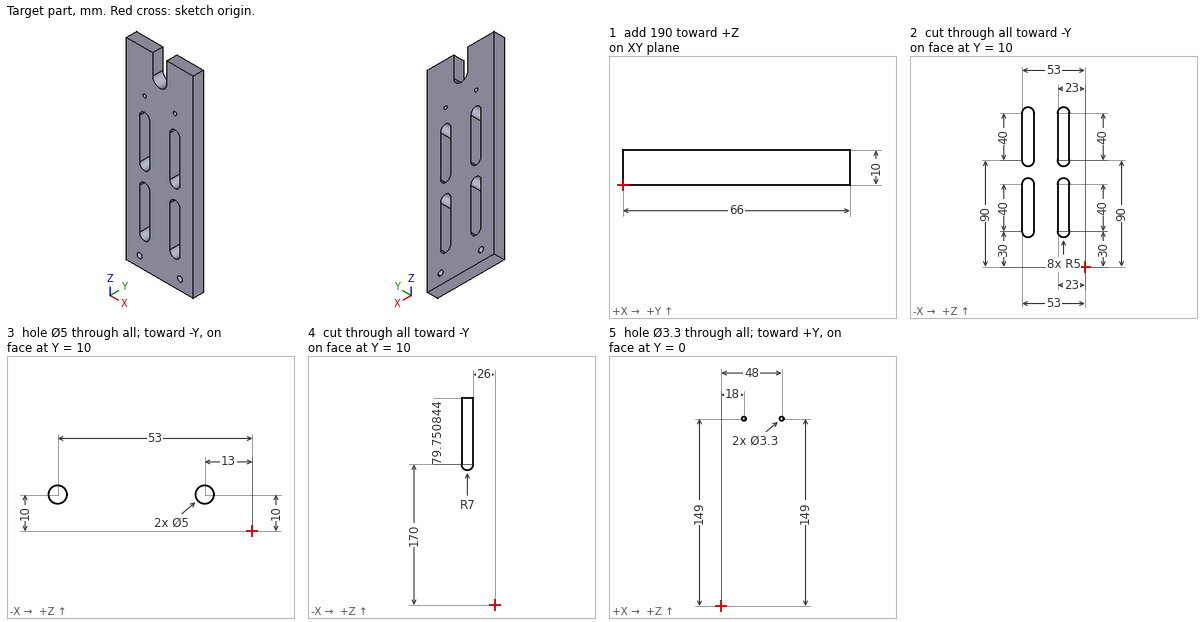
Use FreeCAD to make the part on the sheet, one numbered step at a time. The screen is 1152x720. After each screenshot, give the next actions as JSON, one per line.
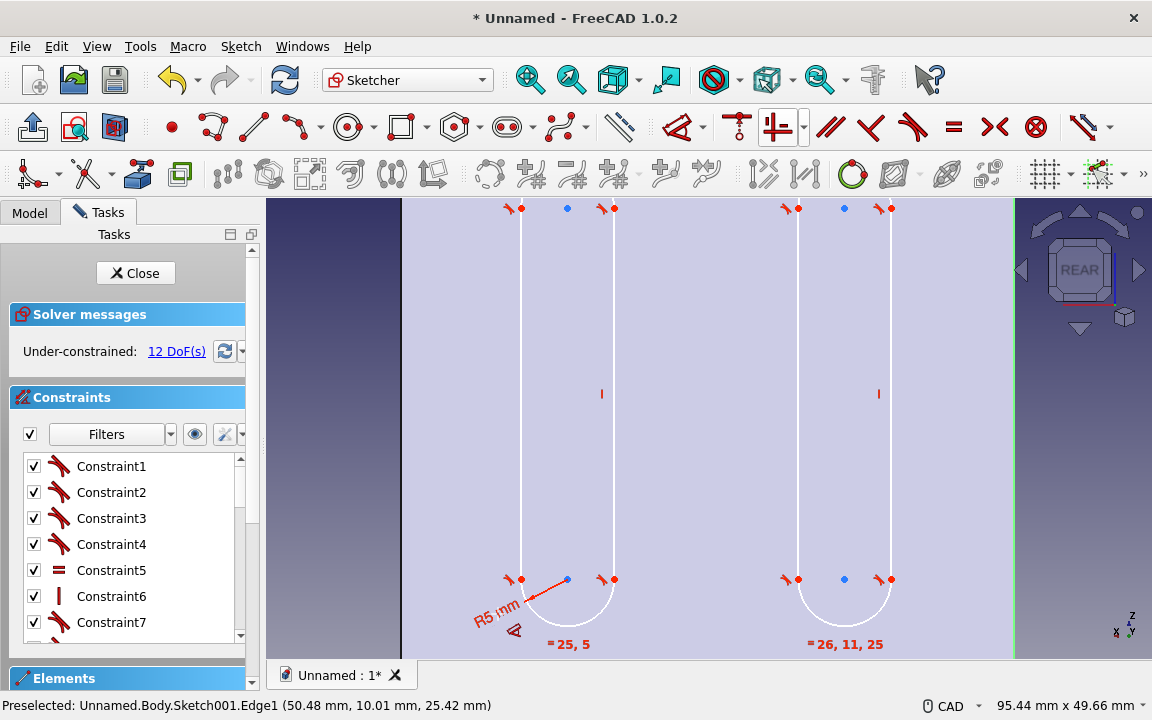
{"action": "scroll", "coordinate": [599, 494], "scroll_direction": "down", "scroll_amount": 7}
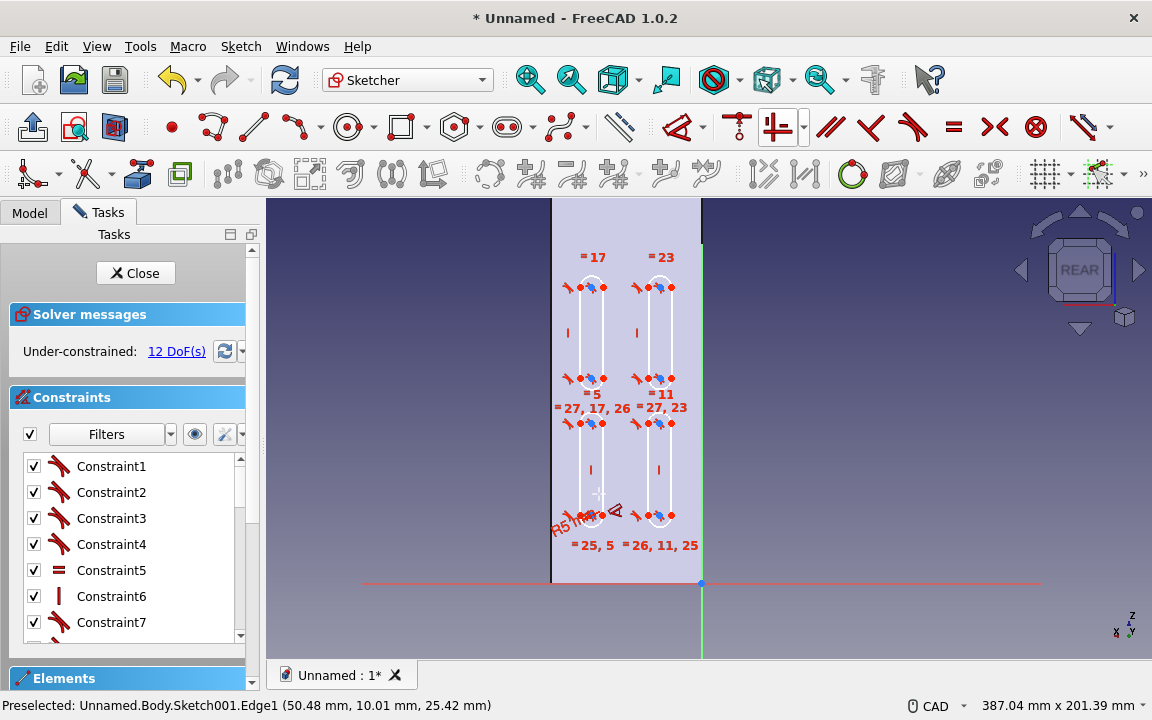
{"action": "left_click", "coordinate": [580, 488]}
{"action": "left_click", "coordinate": [546, 470]}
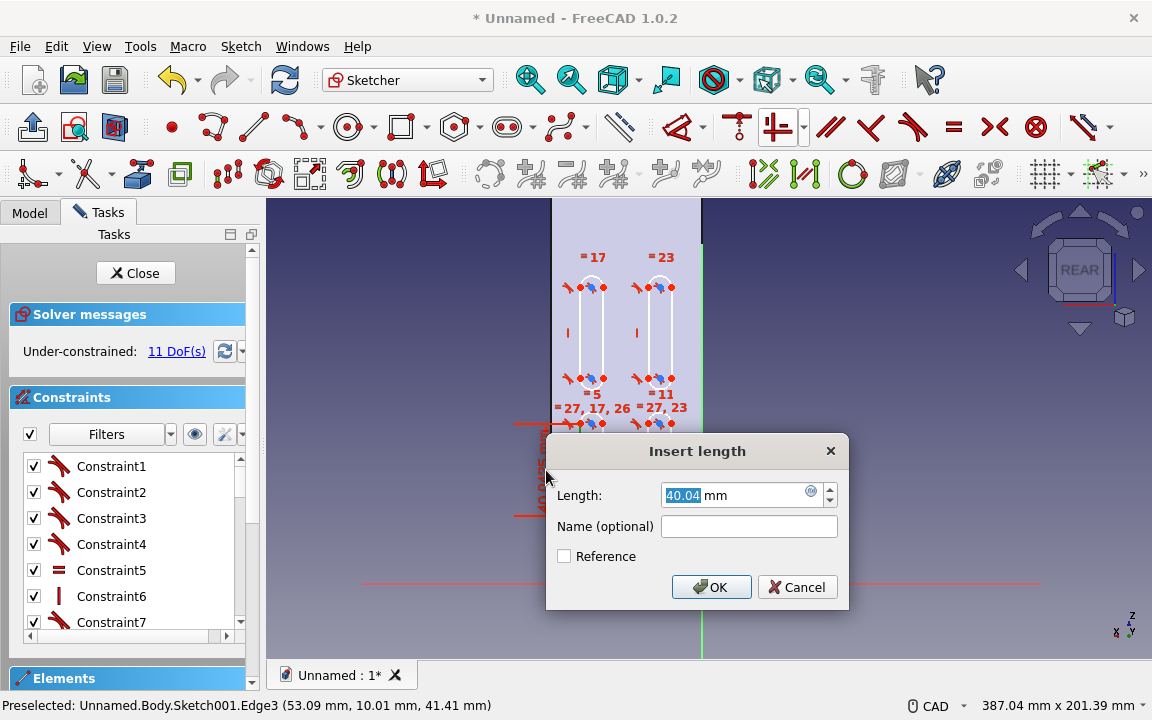
{"action": "type", "text": "40"}
{"action": "key", "text": "Return"}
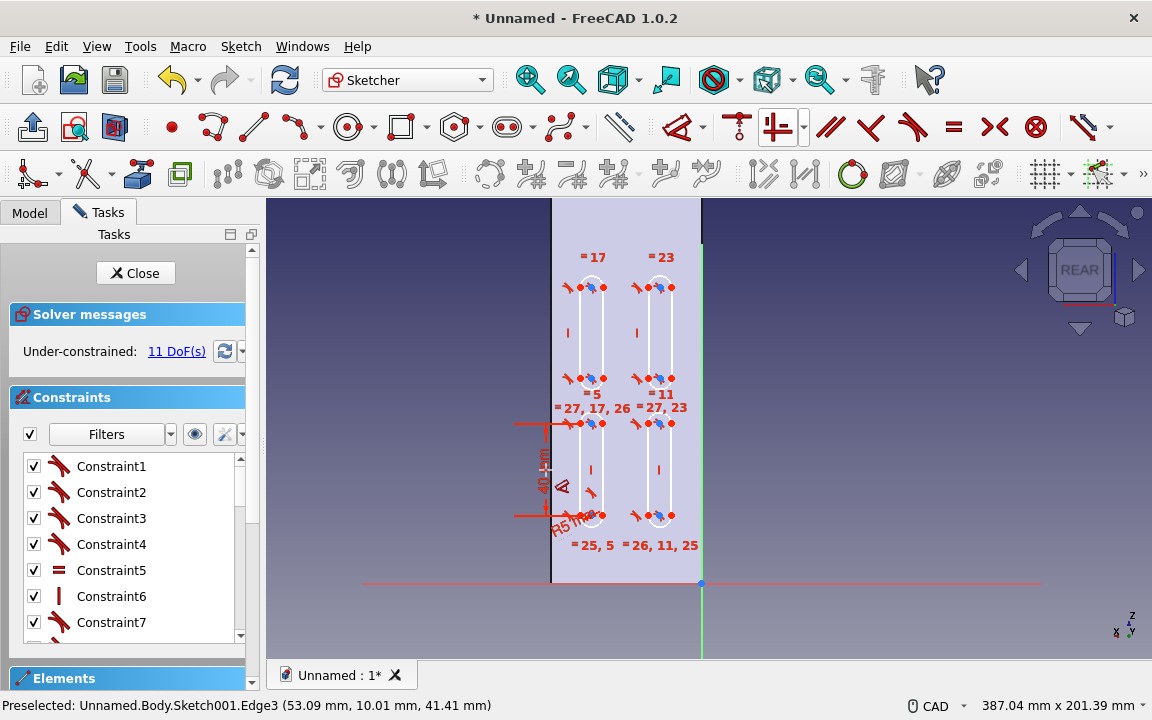
{"action": "left_click", "coordinate": [648, 488]}
{"action": "left_click", "coordinate": [730, 470]}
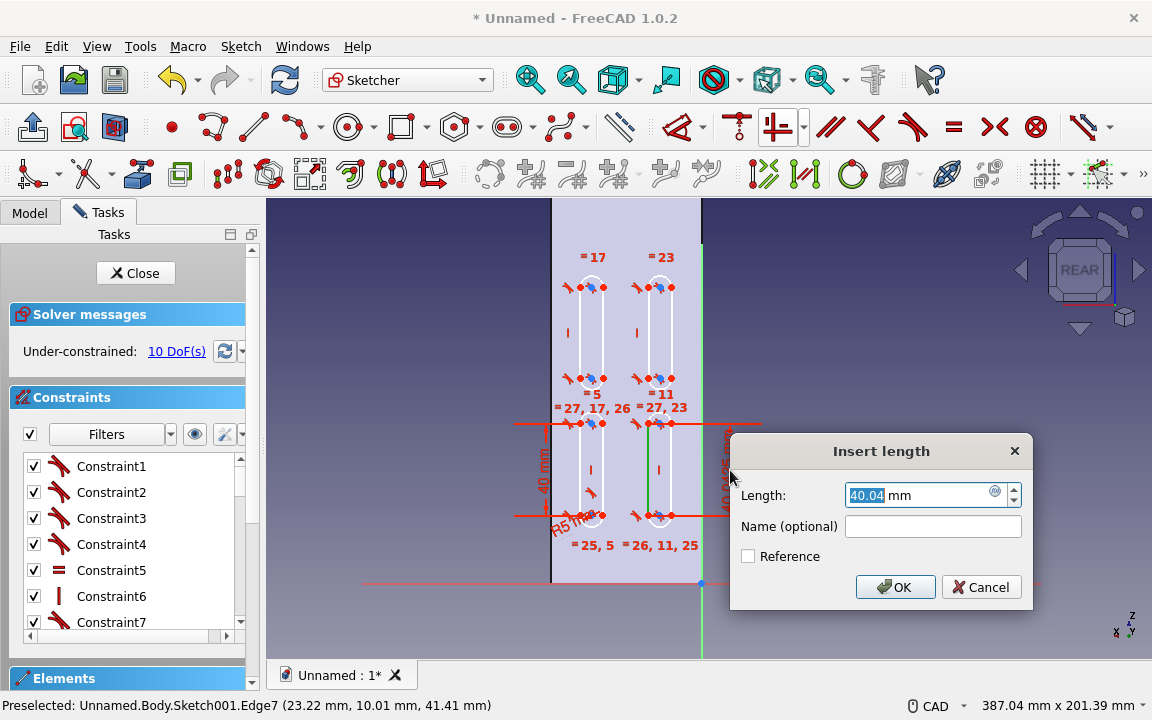
{"action": "type", "text": "40"}
{"action": "key", "text": "Return"}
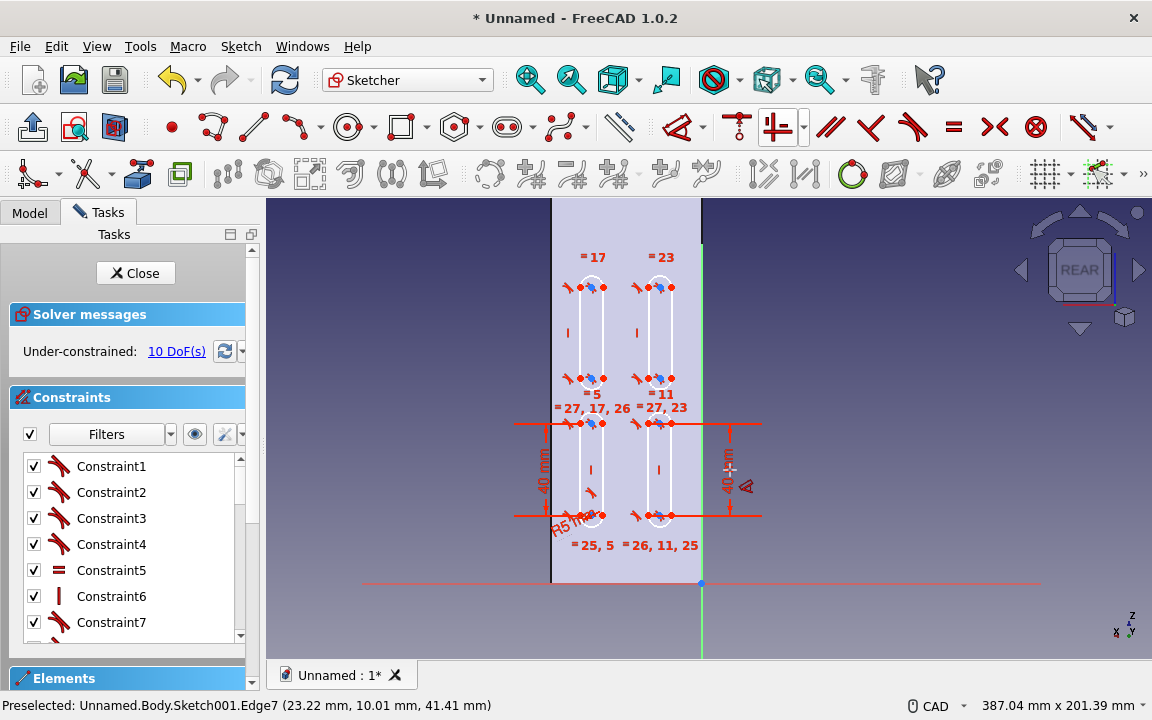
{"action": "left_click", "coordinate": [580, 351]}
{"action": "left_click", "coordinate": [546, 333]}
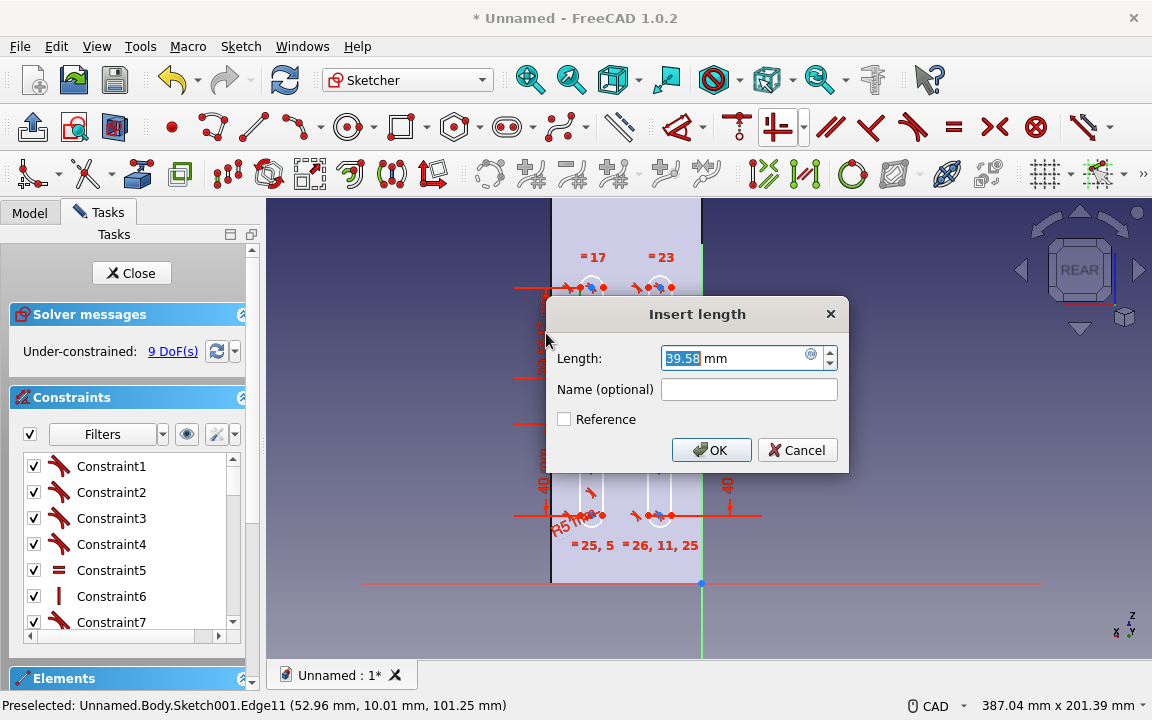
{"action": "type", "text": "40"}
{"action": "key", "text": "Return"}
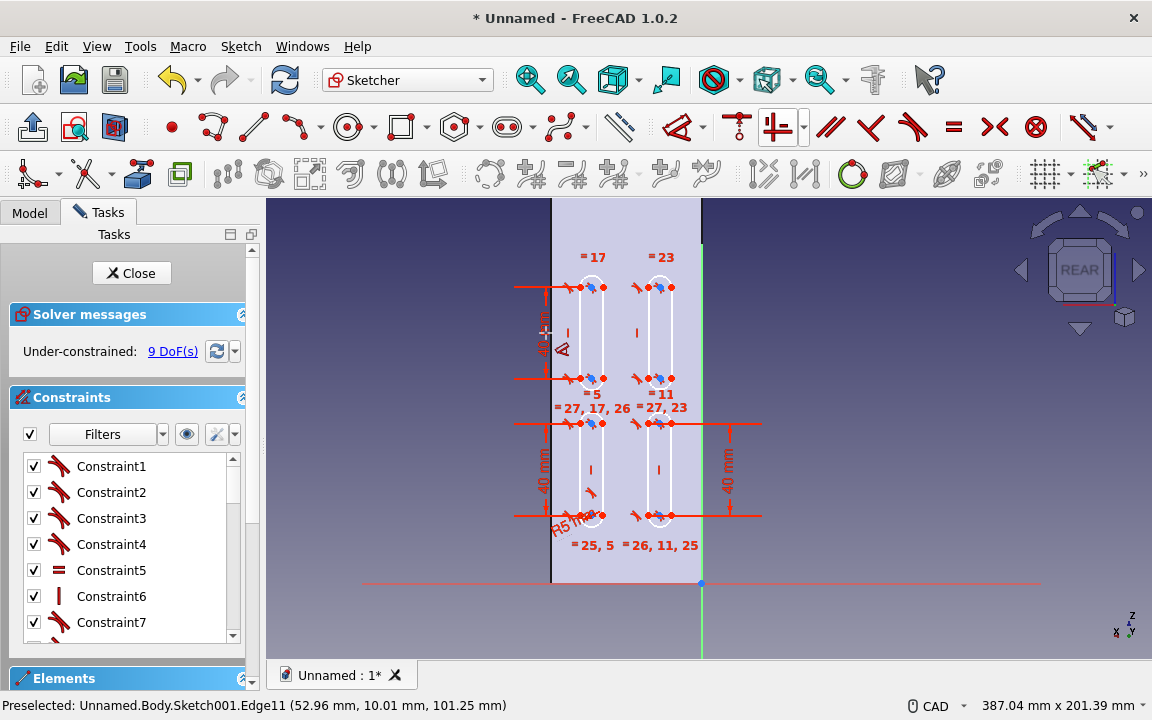
{"action": "left_click", "coordinate": [649, 351]}
{"action": "left_click", "coordinate": [731, 333]}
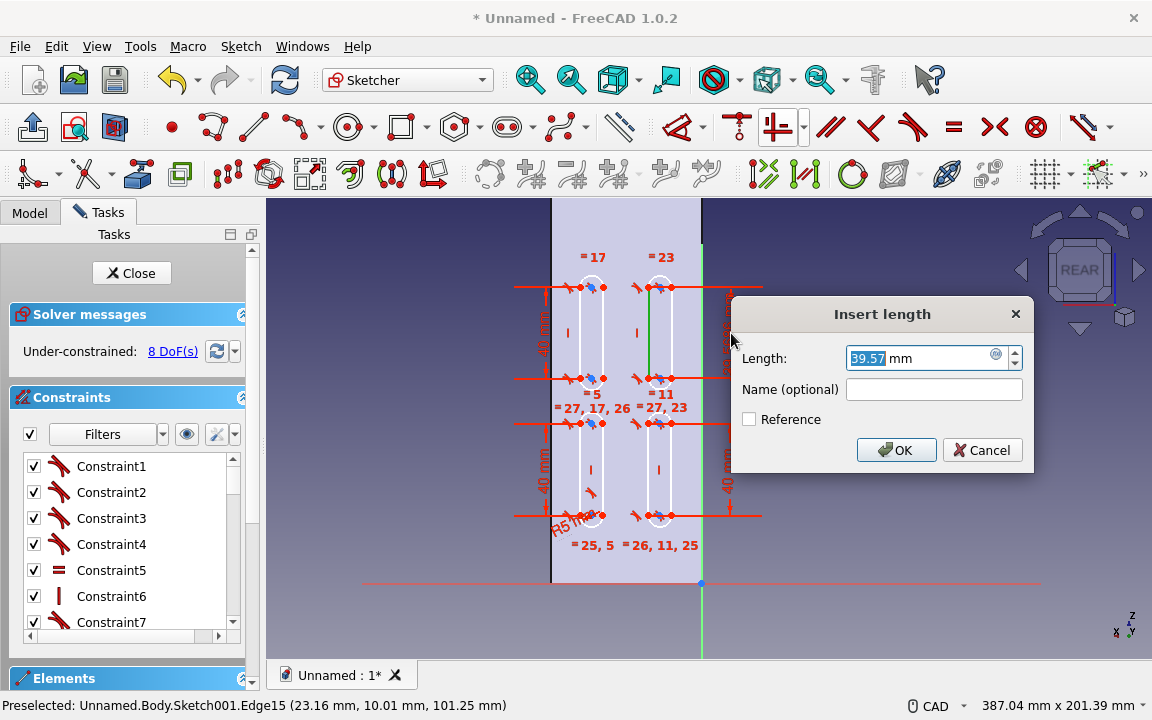
{"action": "type", "text": "40"}
{"action": "key", "text": "Return"}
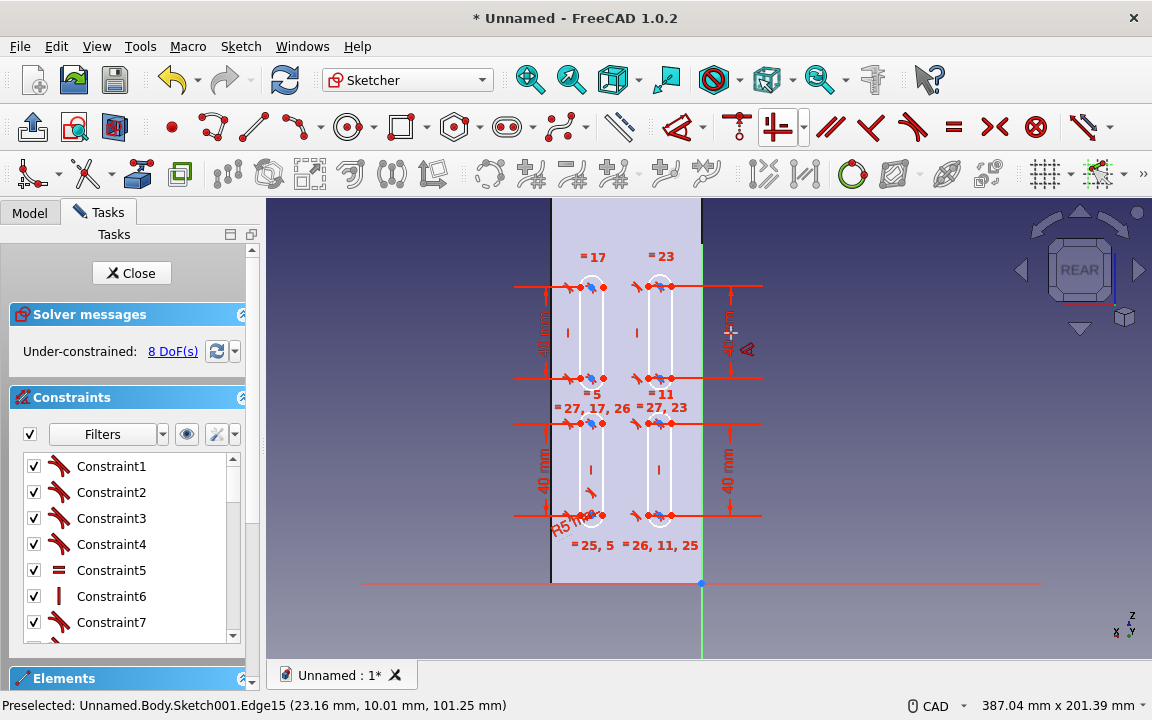
{"action": "left_click", "coordinate": [580, 516]}
{"action": "left_click", "coordinate": [641, 618]}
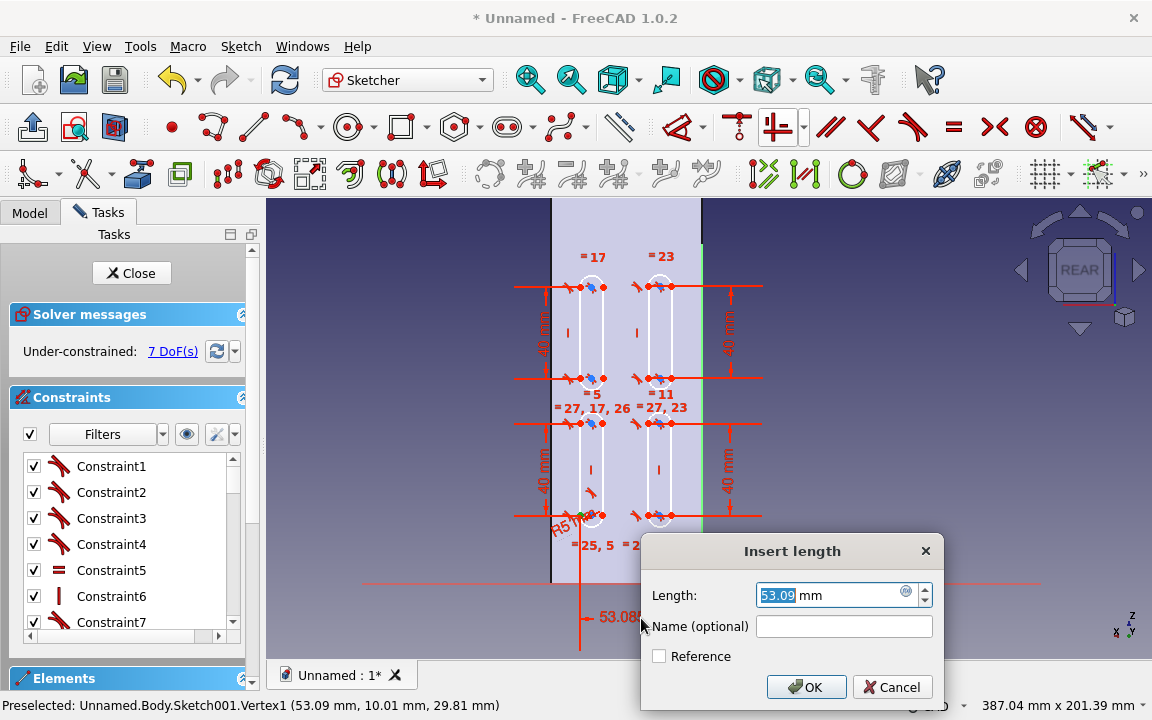
{"action": "type", "text": "53"}
{"action": "key", "text": "Return"}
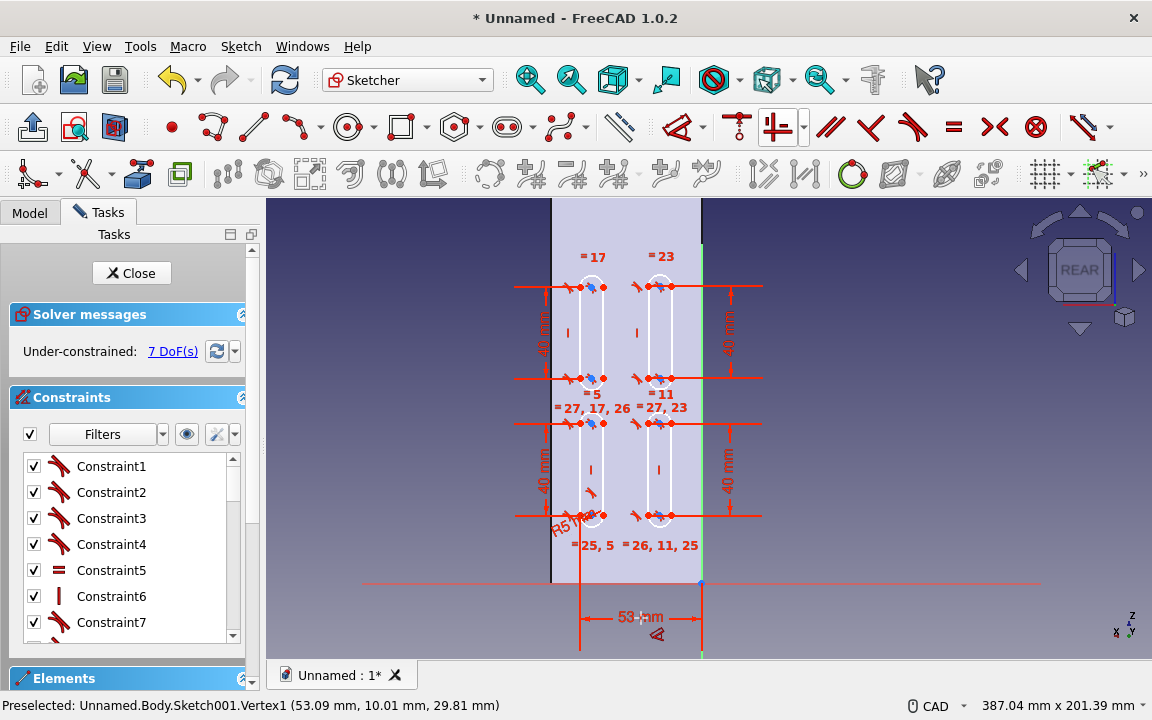
{"action": "left_click", "coordinate": [580, 516]}
{"action": "left_click", "coordinate": [736, 550]}